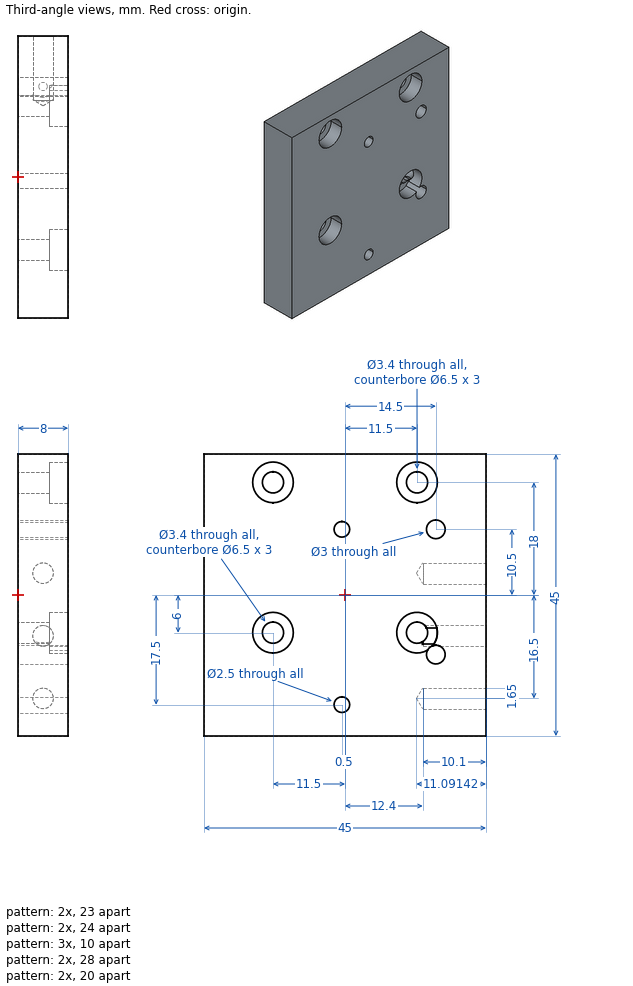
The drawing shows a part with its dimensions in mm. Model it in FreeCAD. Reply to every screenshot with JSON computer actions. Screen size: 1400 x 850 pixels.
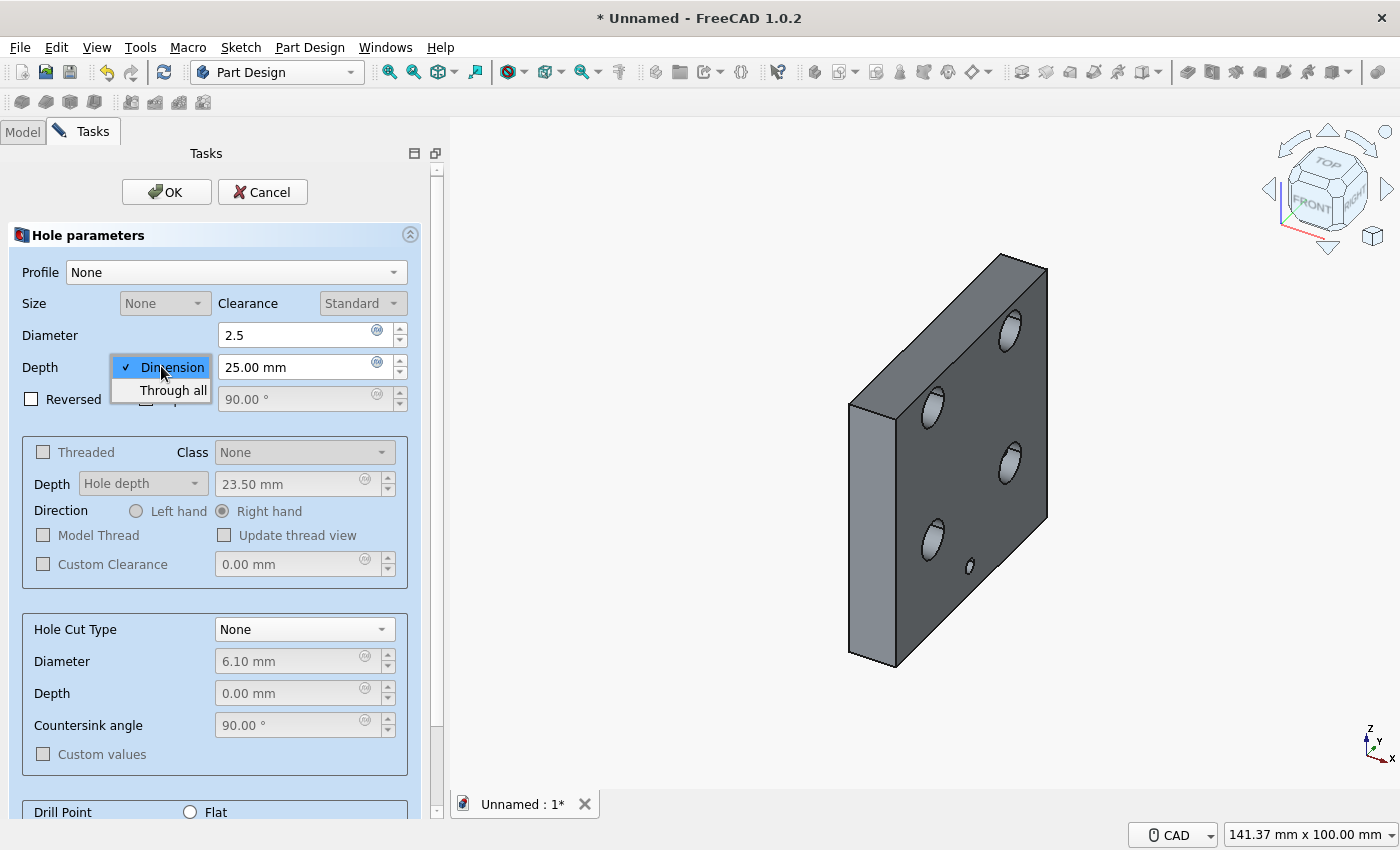
{"action": "left_click", "coordinate": [160, 390]}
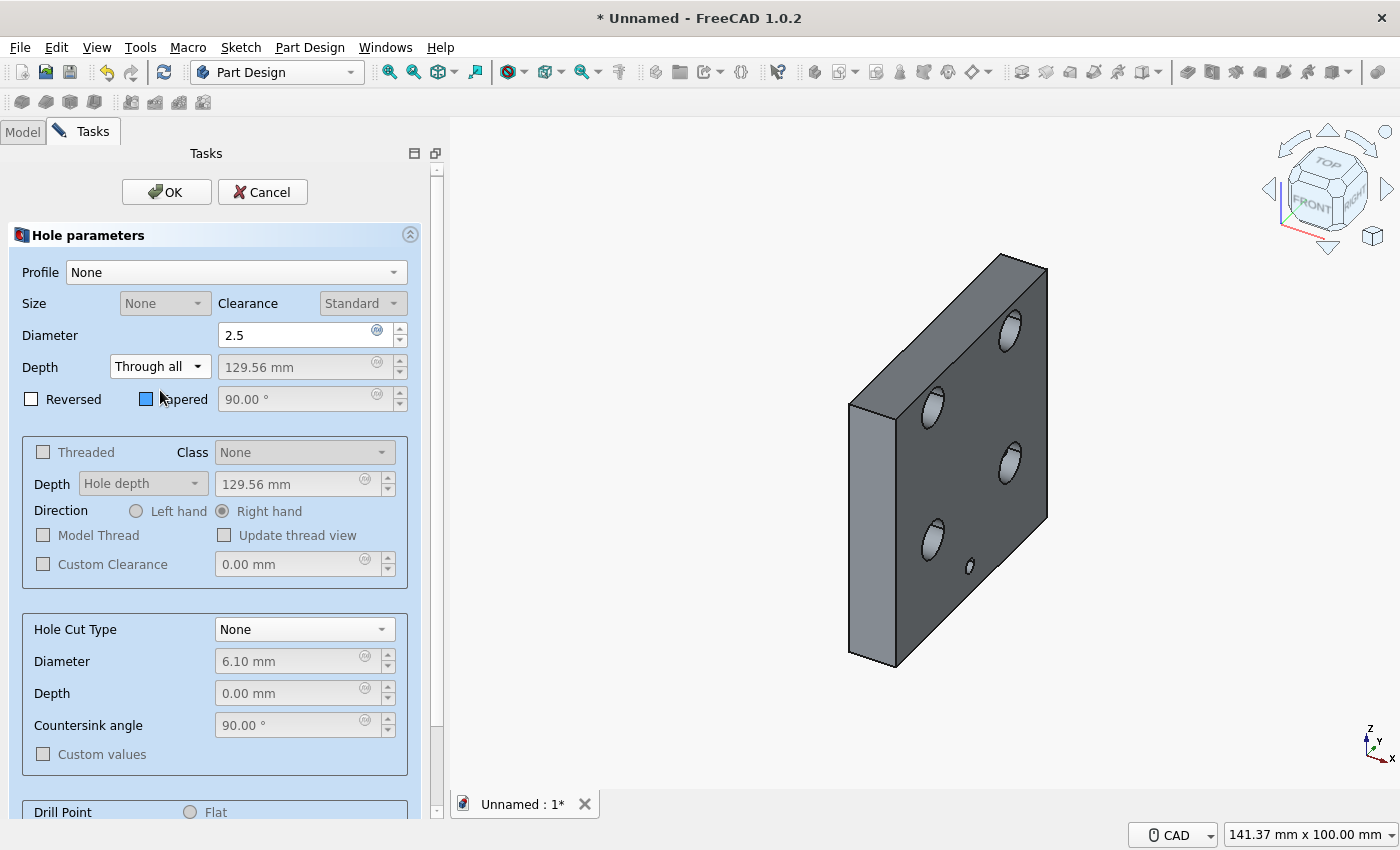
{"action": "left_click", "coordinate": [167, 192]}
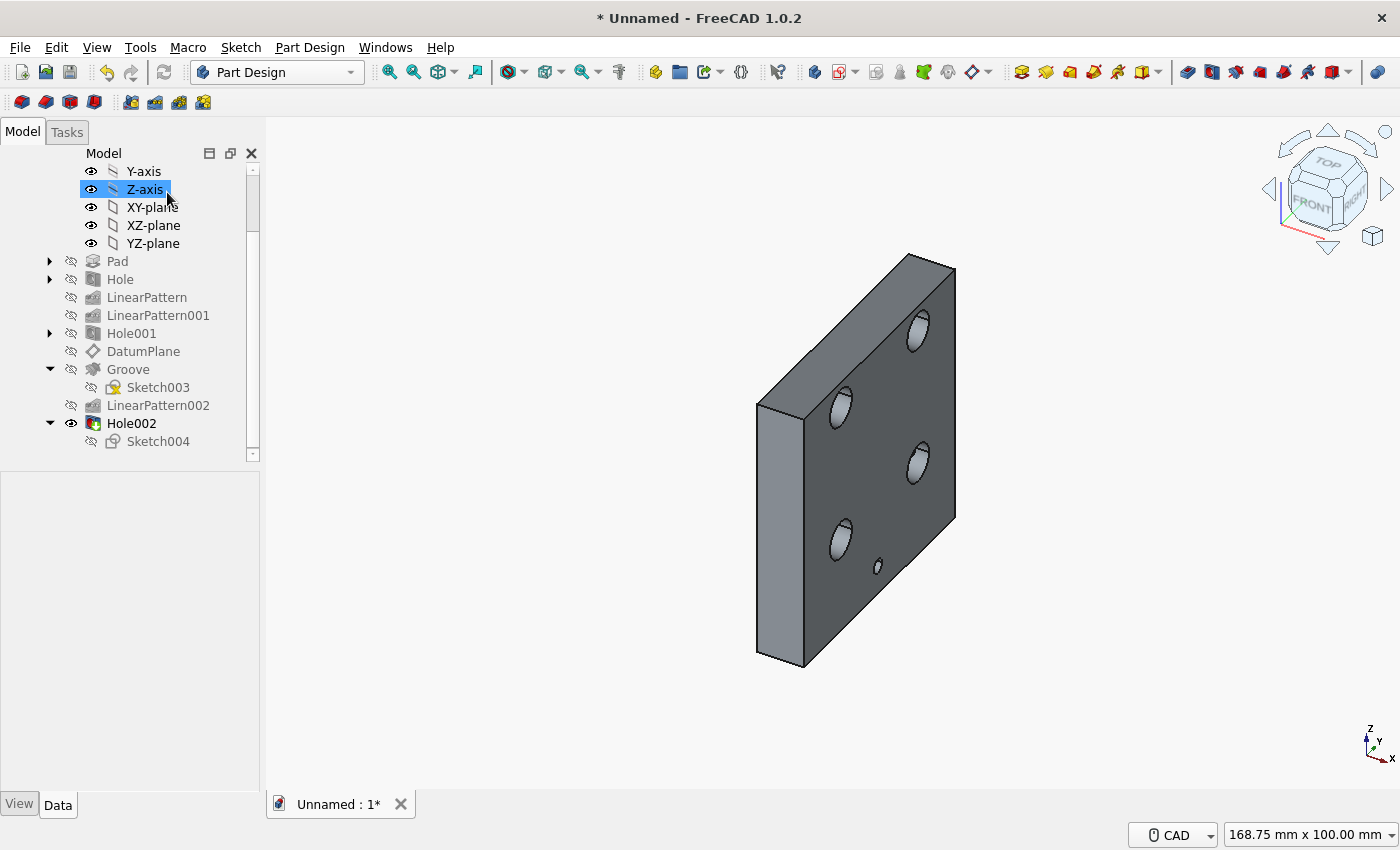
{"action": "left_click", "coordinate": [116, 423]}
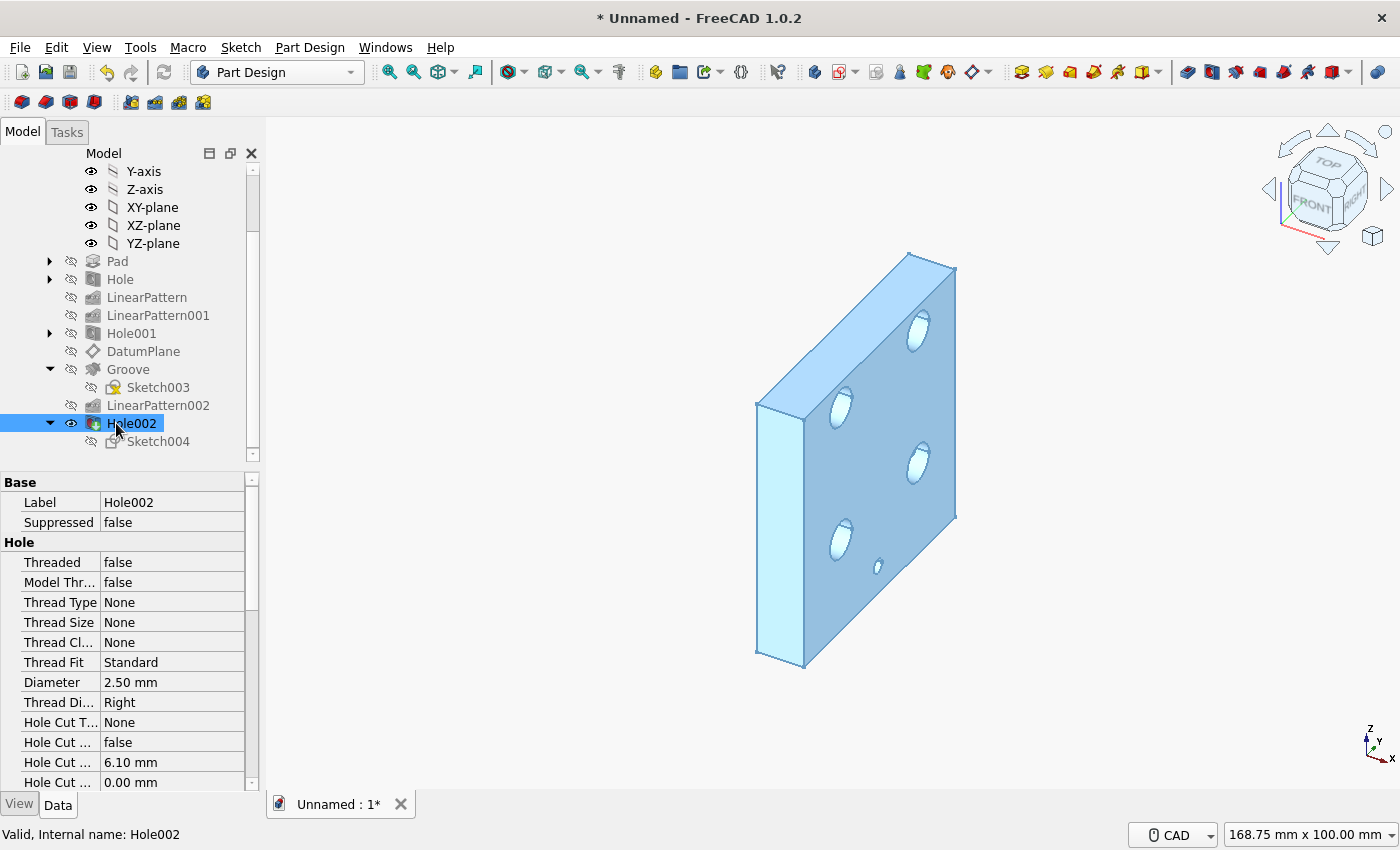
{"action": "left_click", "coordinate": [156, 102]}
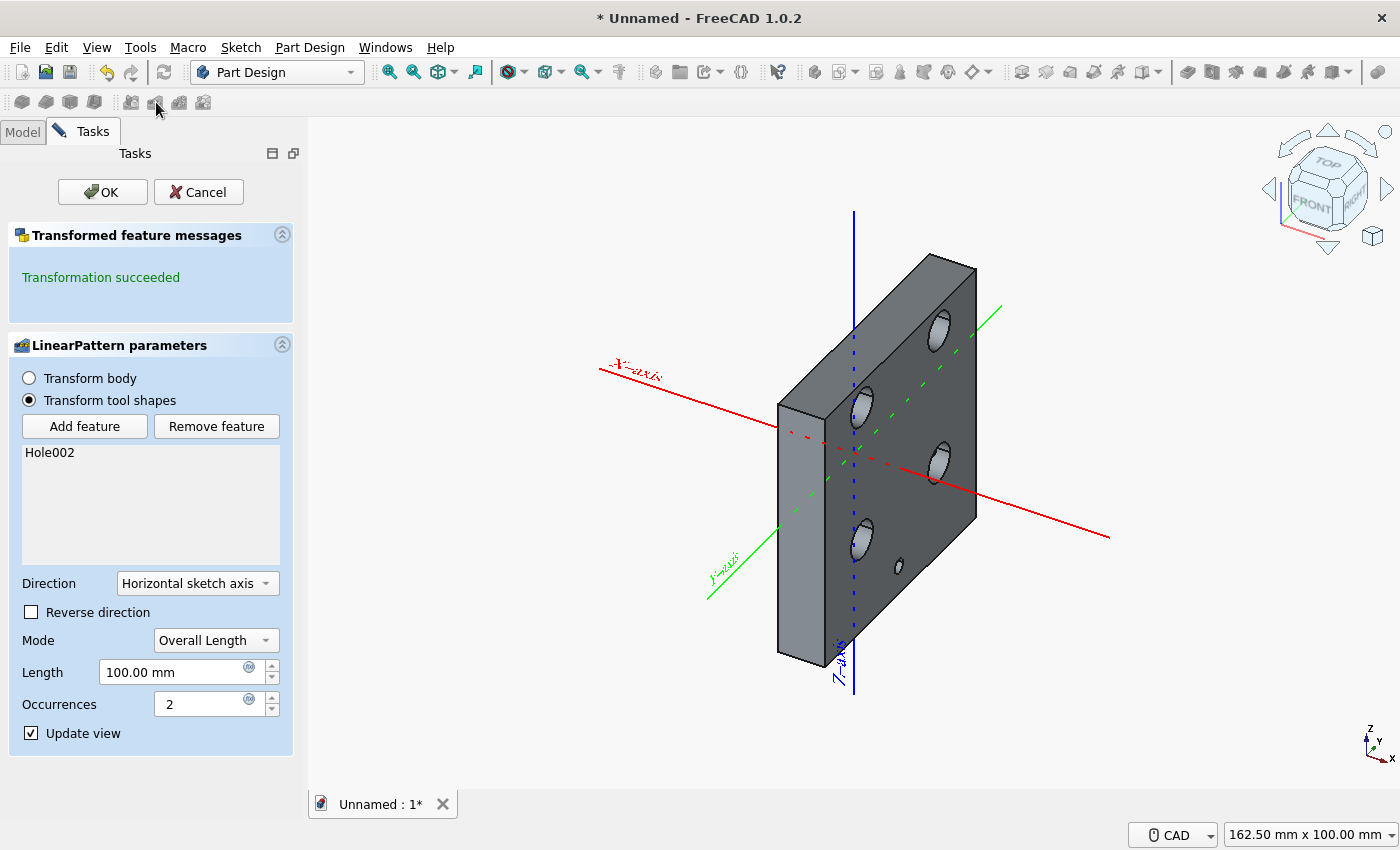
{"action": "left_click", "coordinate": [198, 584]}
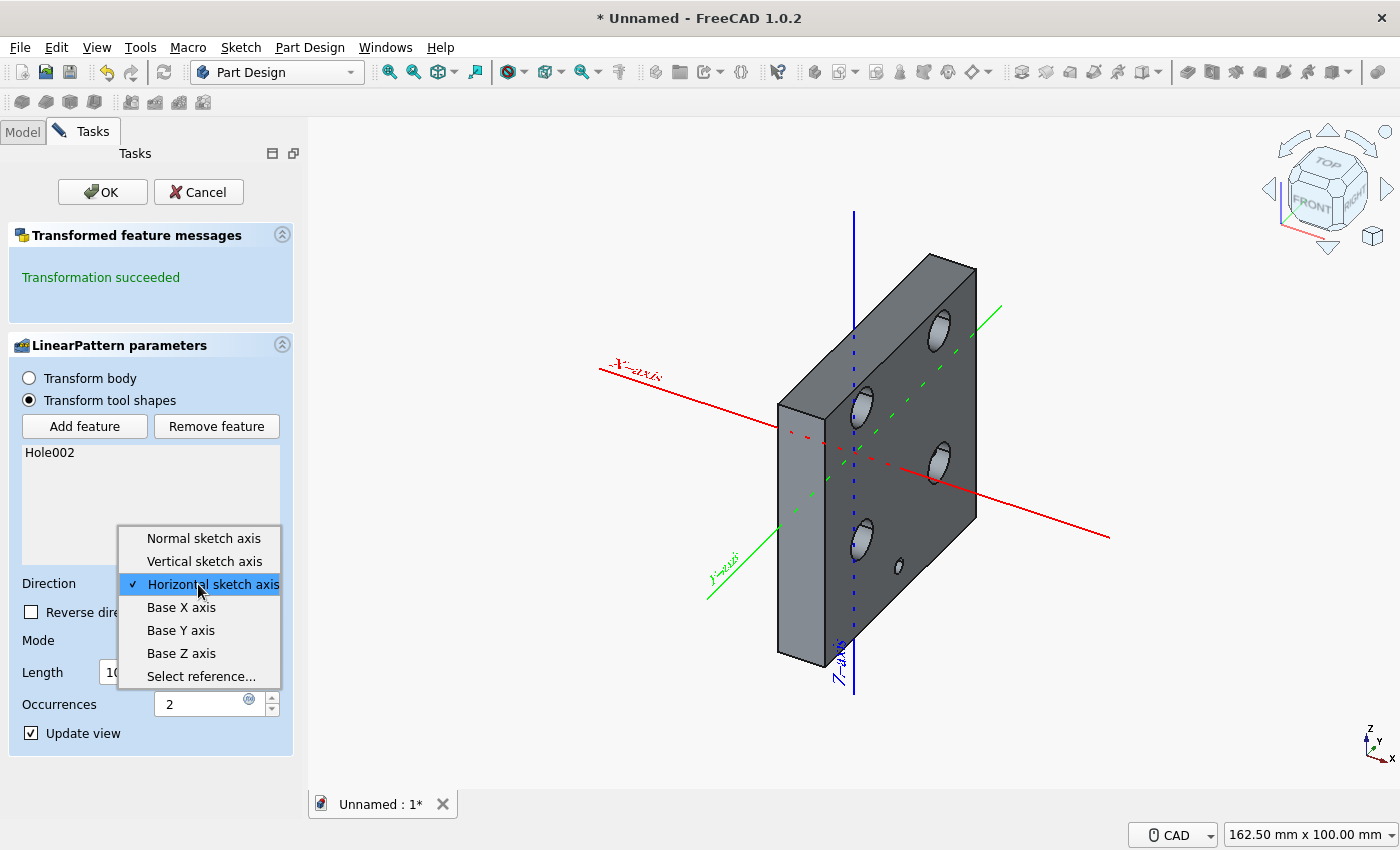
{"action": "left_click", "coordinate": [198, 654]}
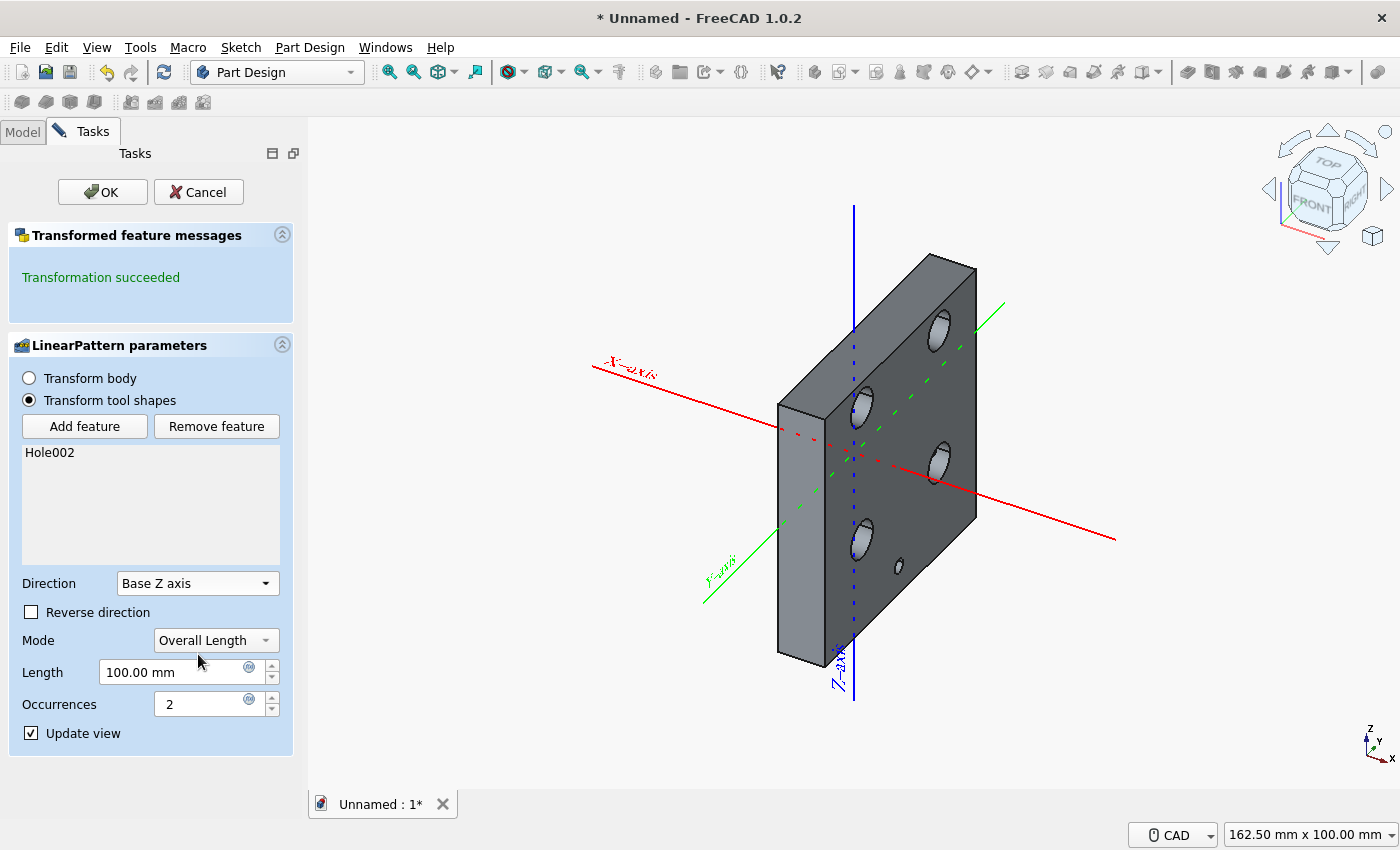
{"action": "left_click", "coordinate": [217, 640]}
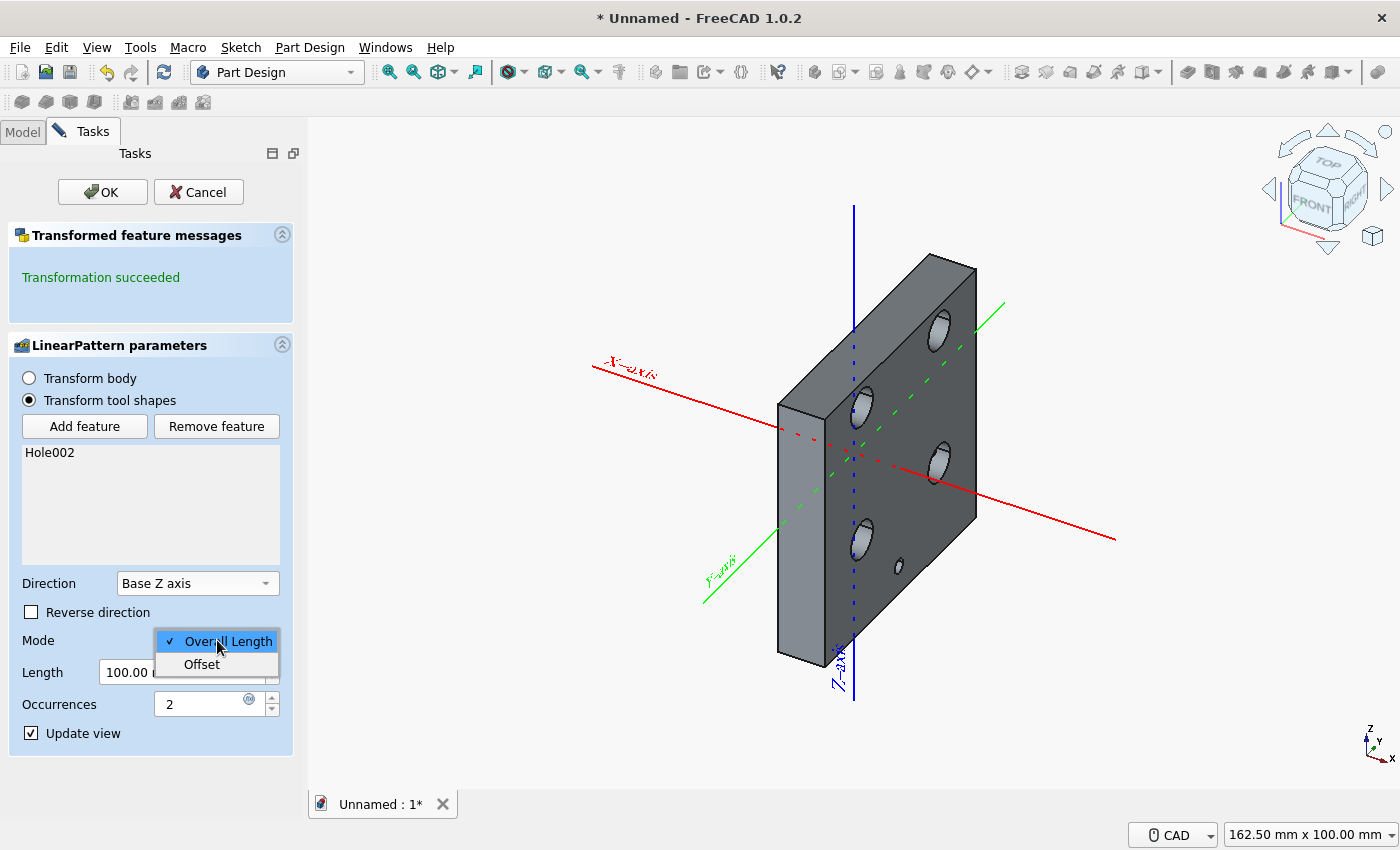
{"action": "left_click", "coordinate": [216, 664]}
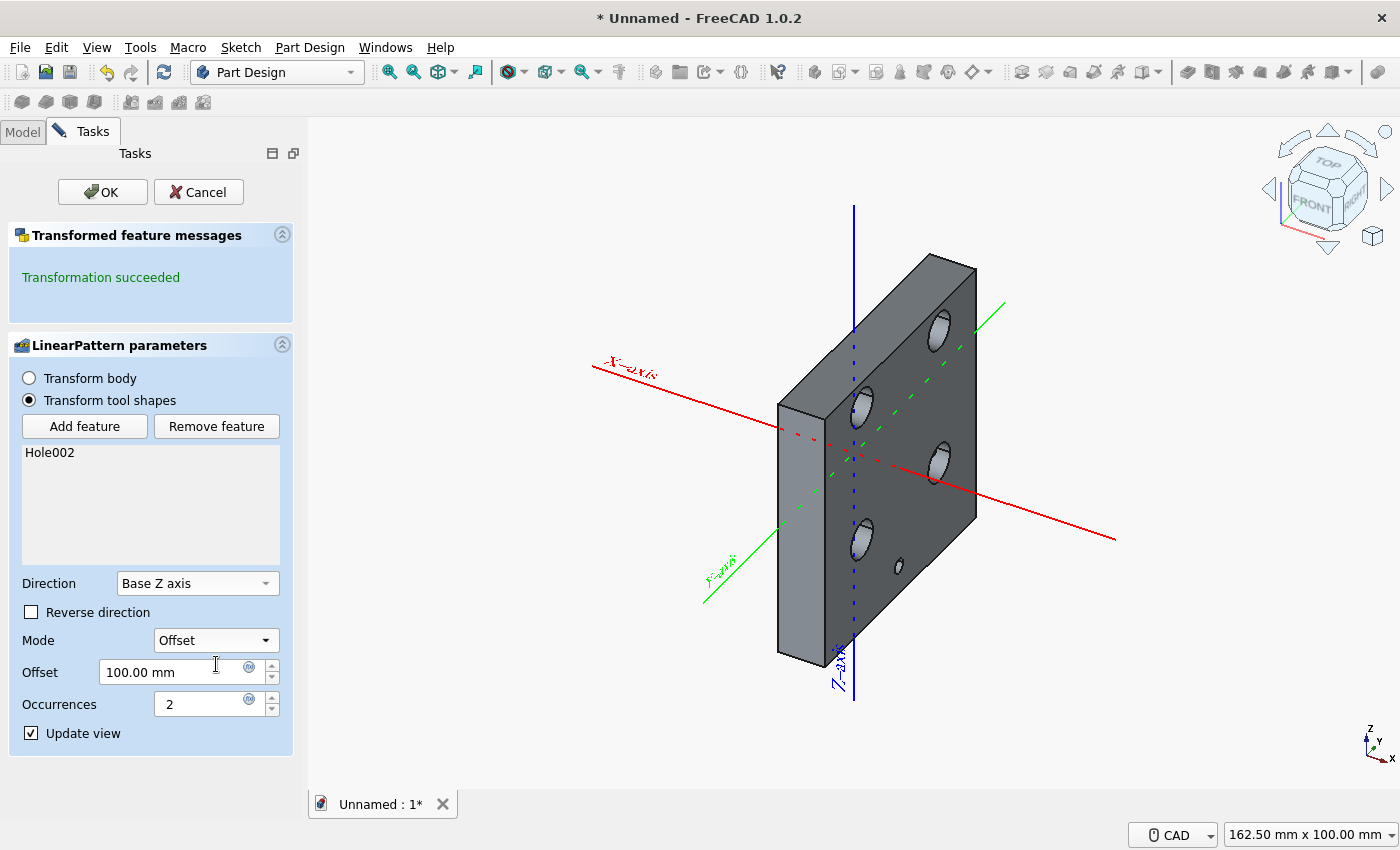
{"action": "triple_click", "coordinate": [182, 672]}